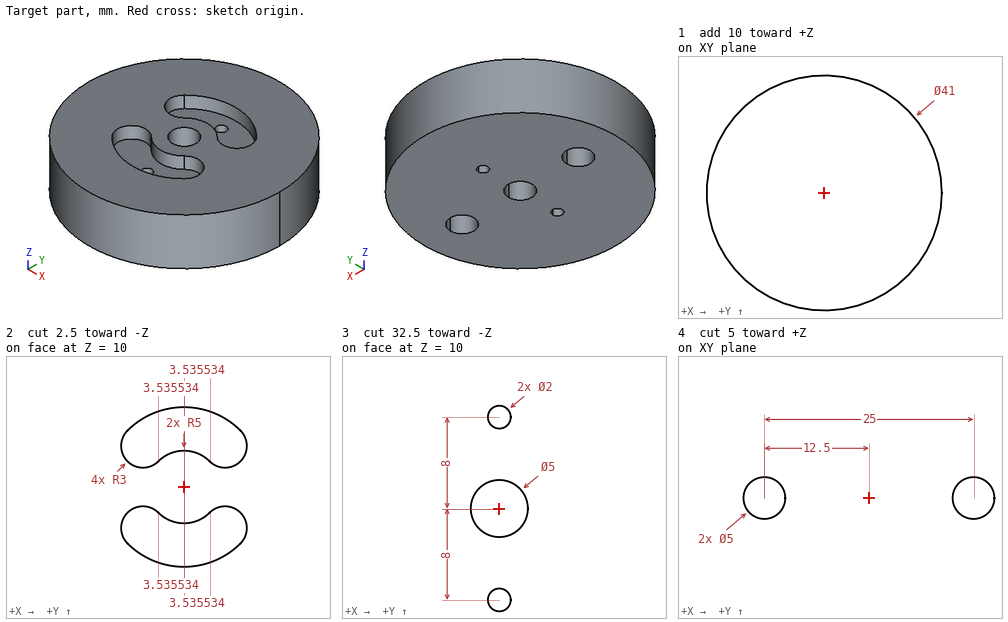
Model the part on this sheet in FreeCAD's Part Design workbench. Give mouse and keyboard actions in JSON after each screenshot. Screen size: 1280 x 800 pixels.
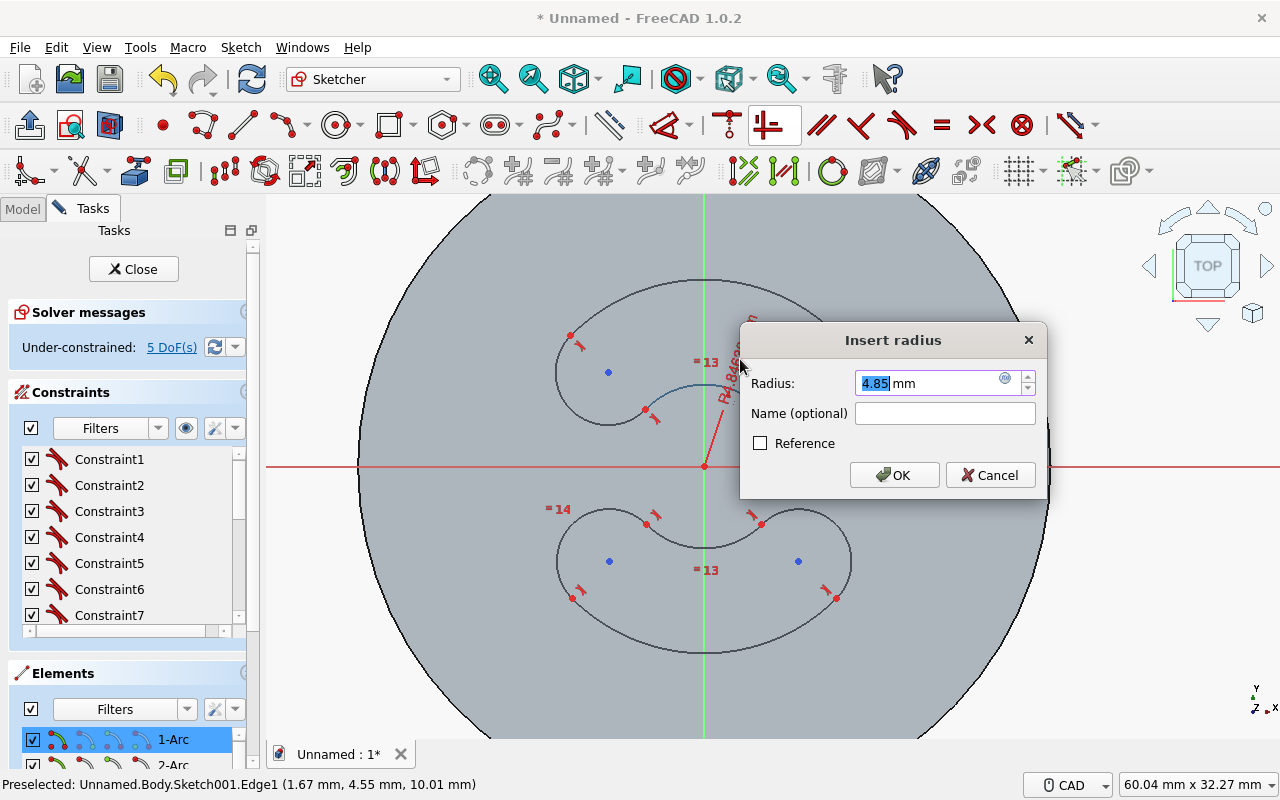
{"action": "type", "text": "5"}
{"action": "key", "text": "Return"}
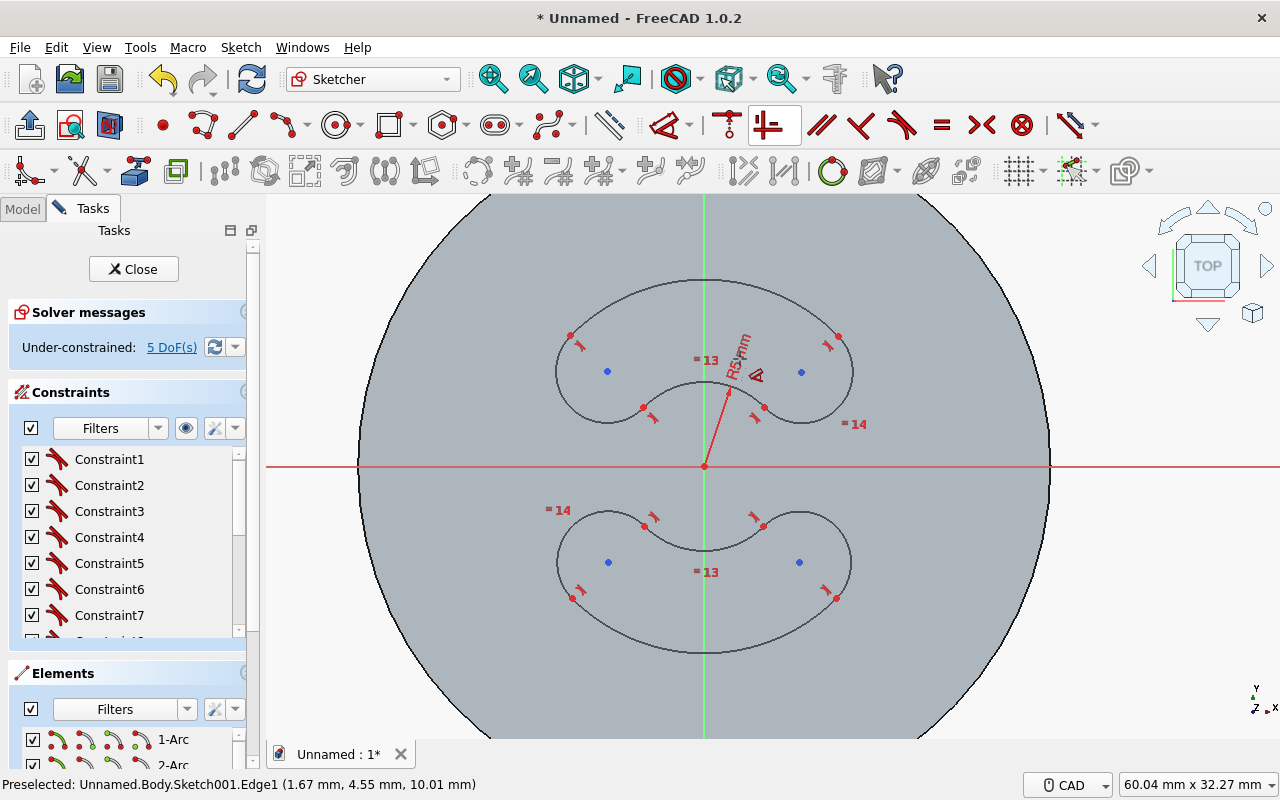
{"action": "left_click", "coordinate": [809, 423]}
{"action": "left_click", "coordinate": [773, 450]}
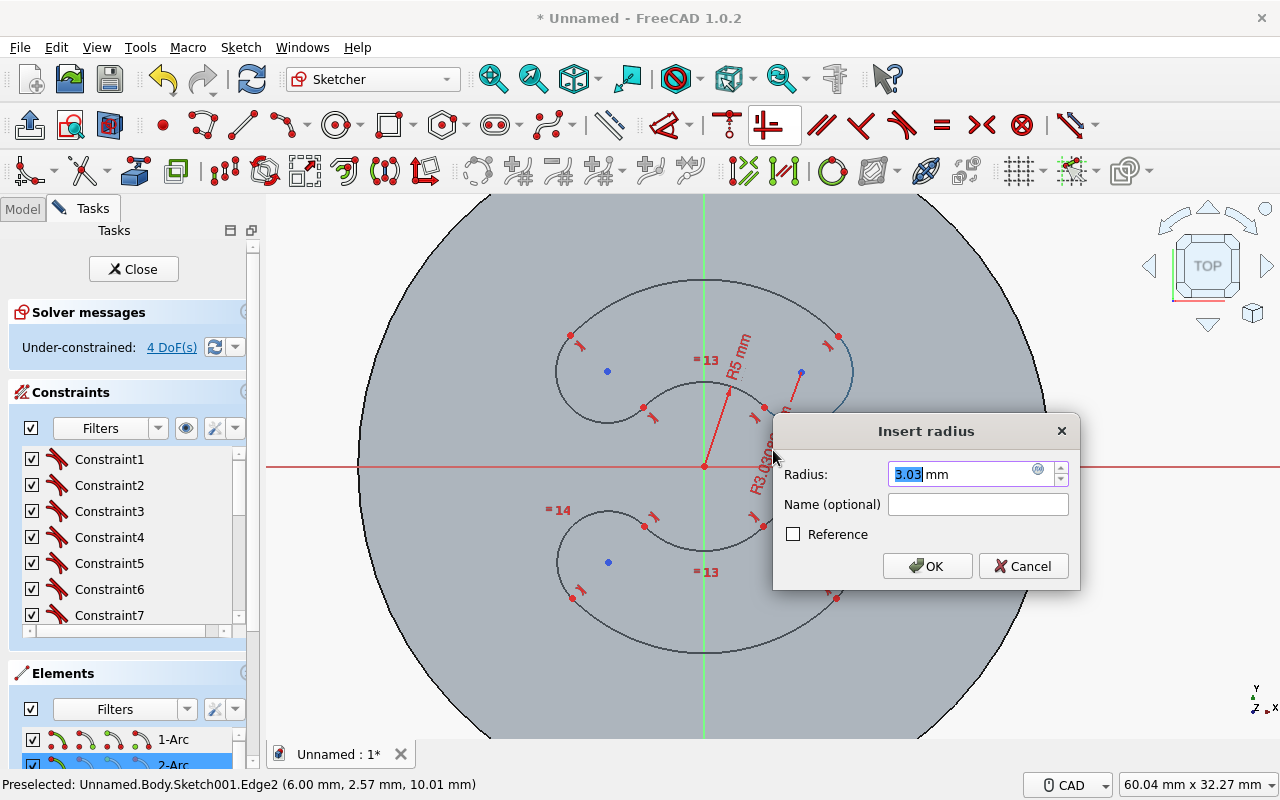
{"action": "type", "text": "3"}
{"action": "key", "text": "Return"}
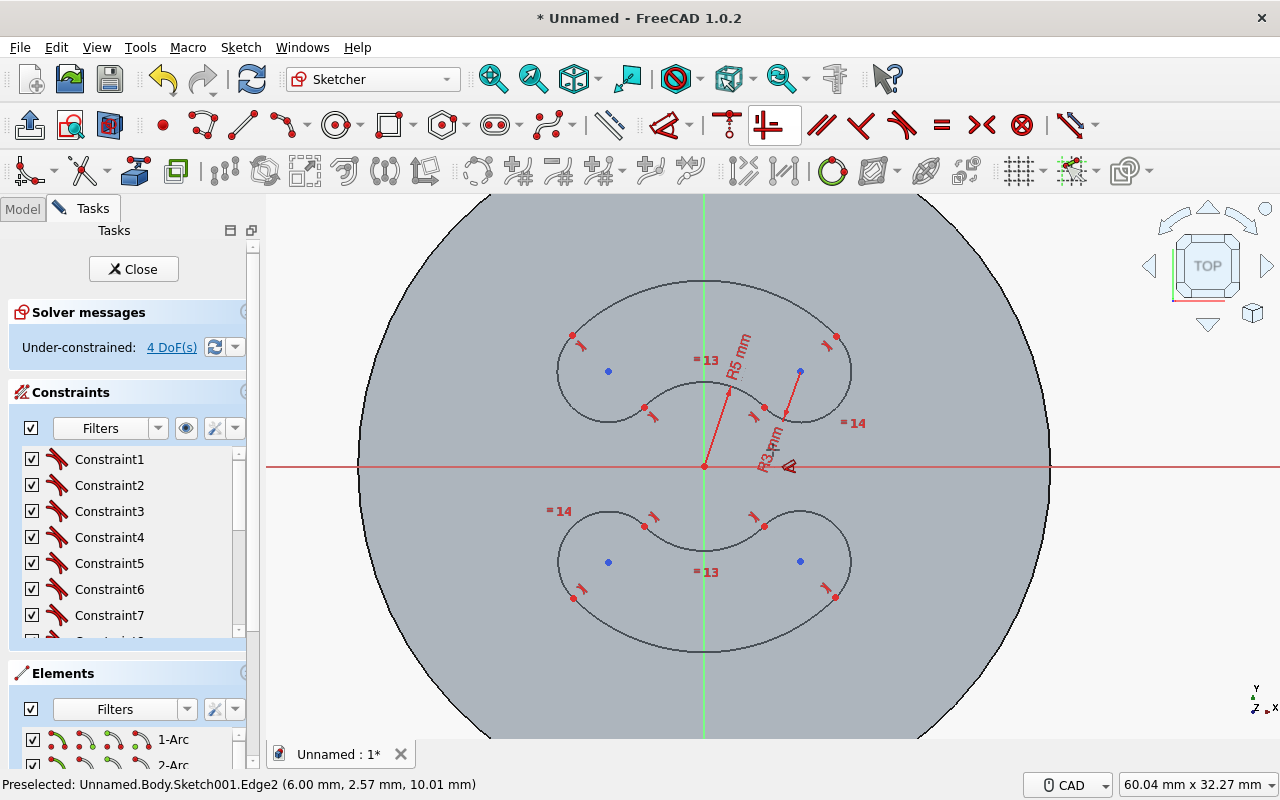
{"action": "left_click", "coordinate": [765, 407]}
{"action": "left_click", "coordinate": [734, 500]}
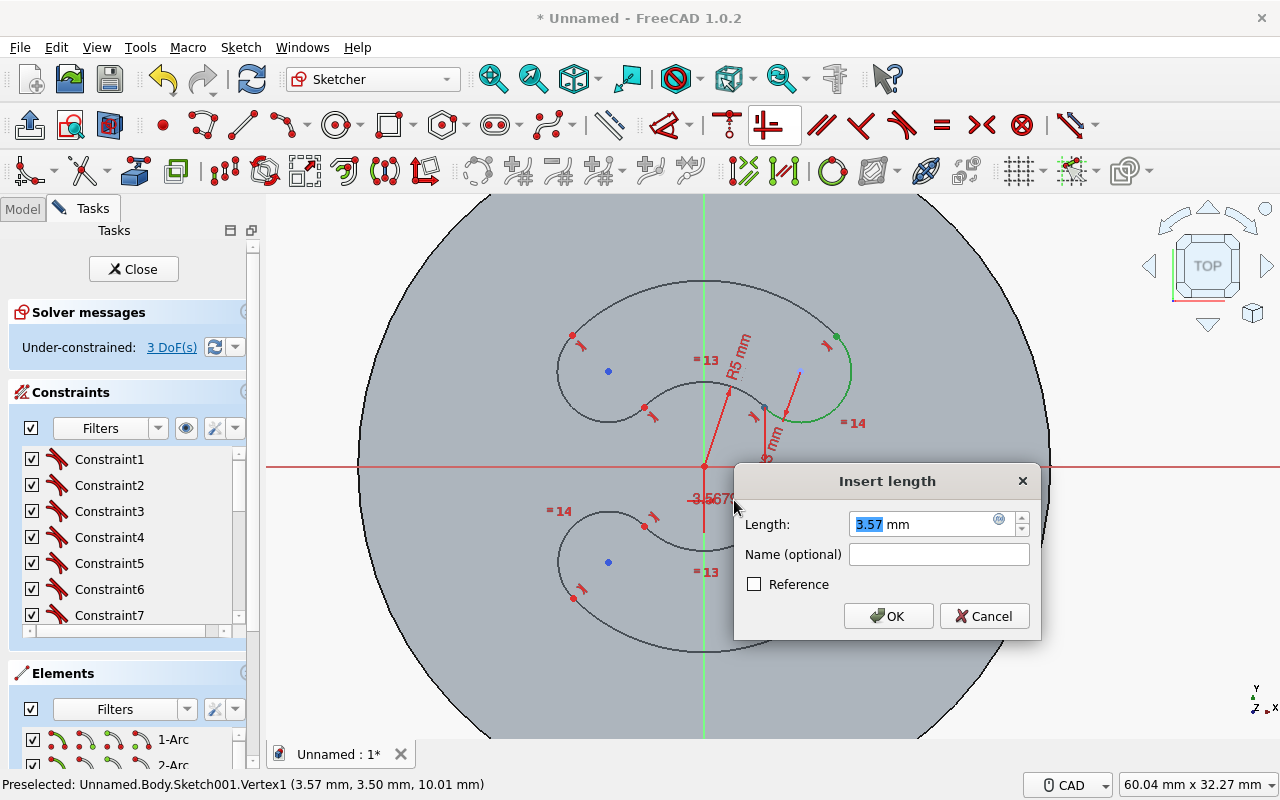
{"action": "type", "text": "3.535534"}
{"action": "key", "text": "Return"}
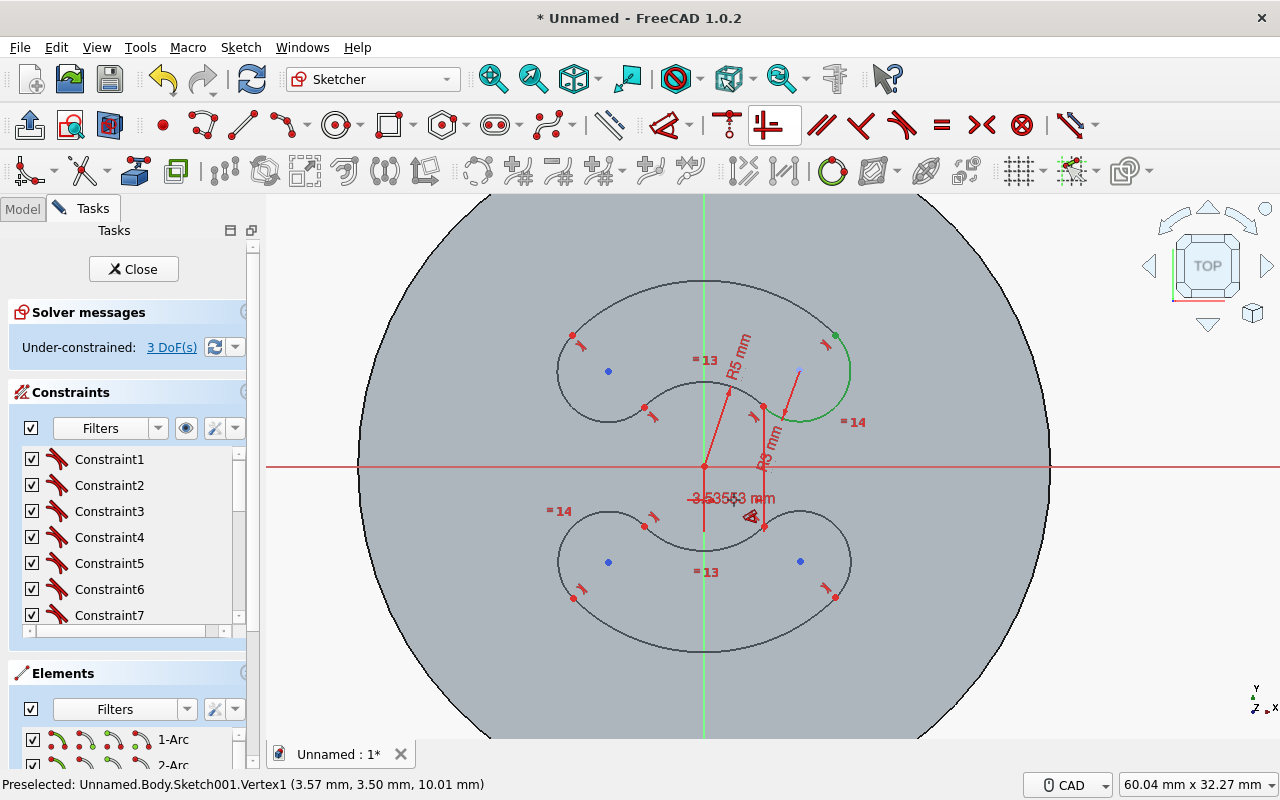
{"action": "left_click", "coordinate": [644, 407]}
{"action": "left_click", "coordinate": [660, 373]}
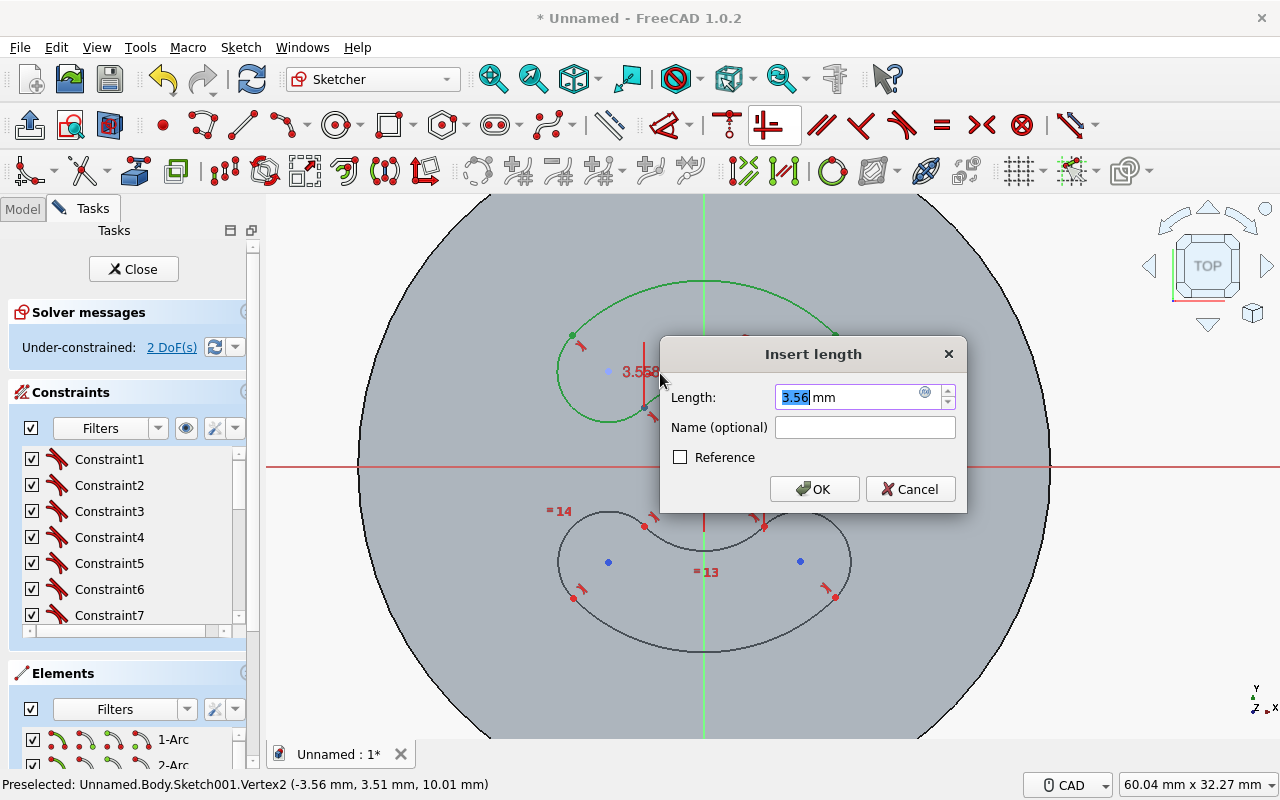
{"action": "type", "text": "3.535534"}
{"action": "key", "text": "Return"}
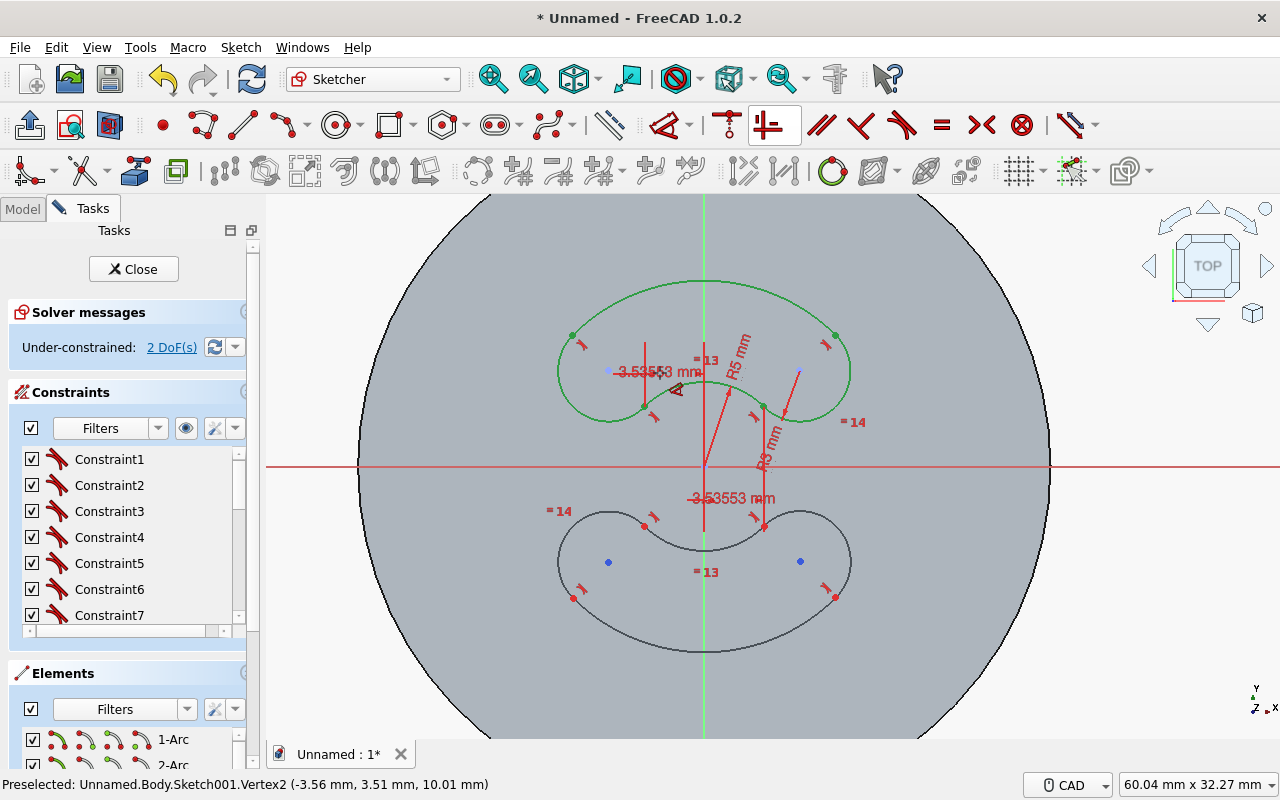
{"action": "left_click", "coordinate": [645, 526]}
{"action": "left_click", "coordinate": [674, 560]}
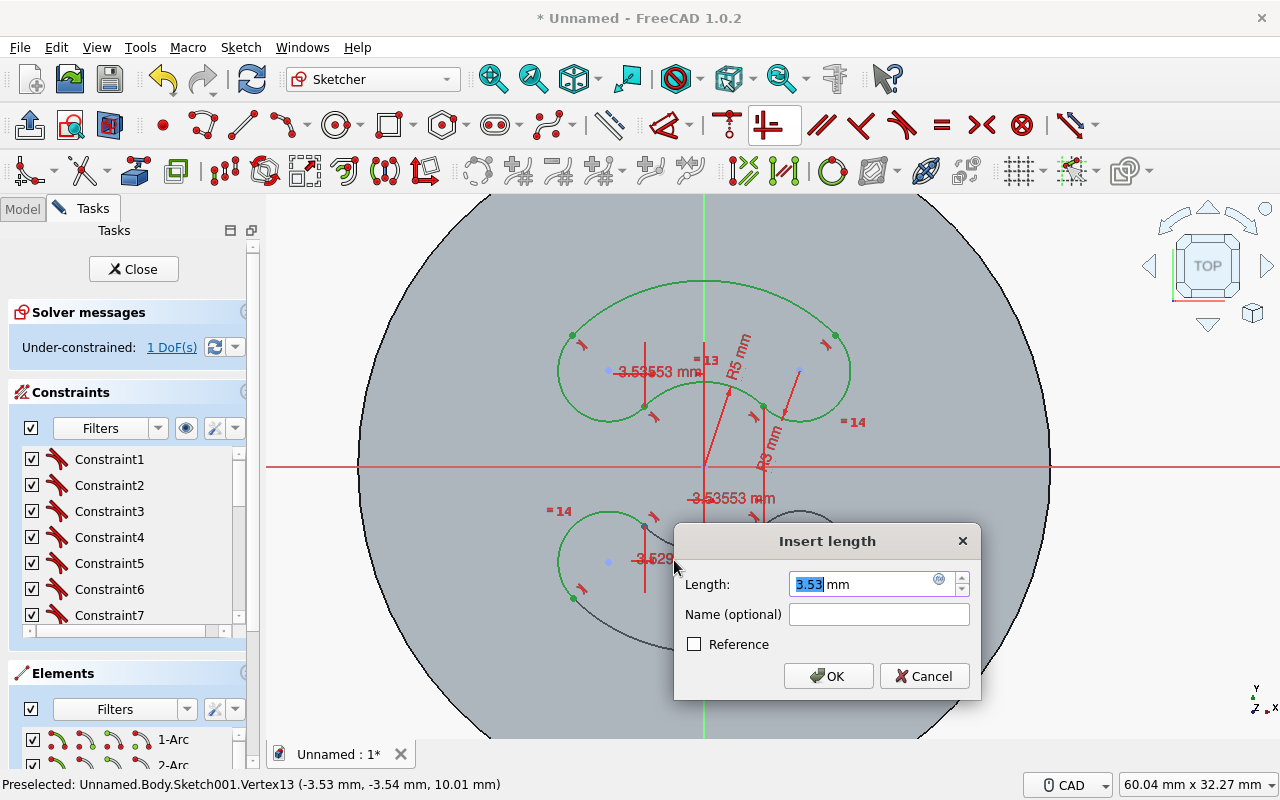
{"action": "type", "text": "3.535534"}
{"action": "key", "text": "Return"}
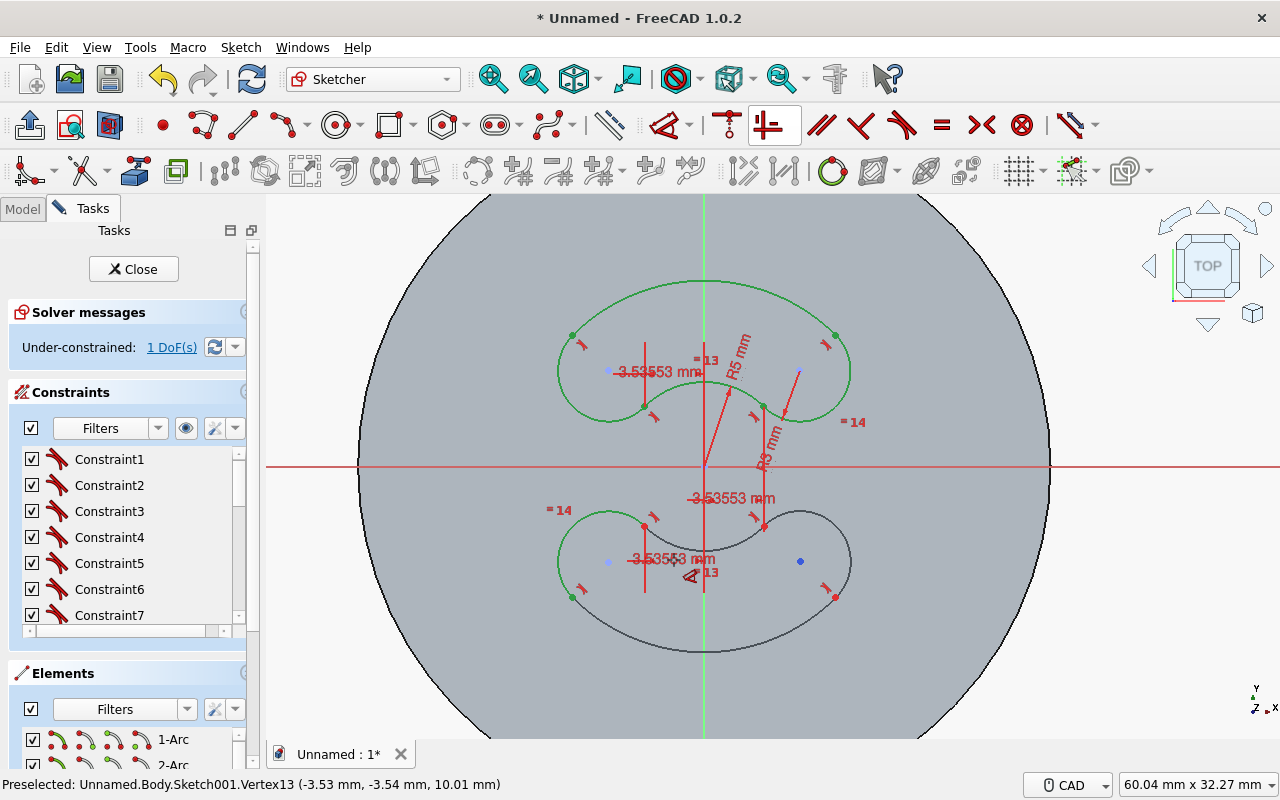
{"action": "left_click", "coordinate": [764, 526]}
{"action": "left_click", "coordinate": [748, 560]}